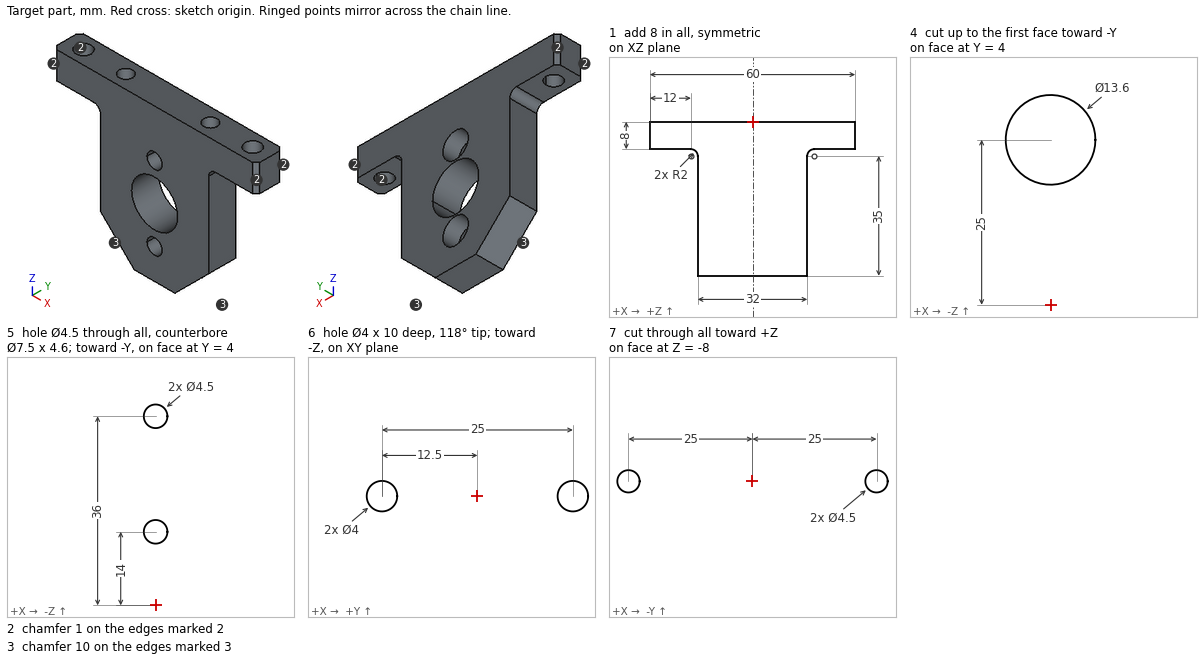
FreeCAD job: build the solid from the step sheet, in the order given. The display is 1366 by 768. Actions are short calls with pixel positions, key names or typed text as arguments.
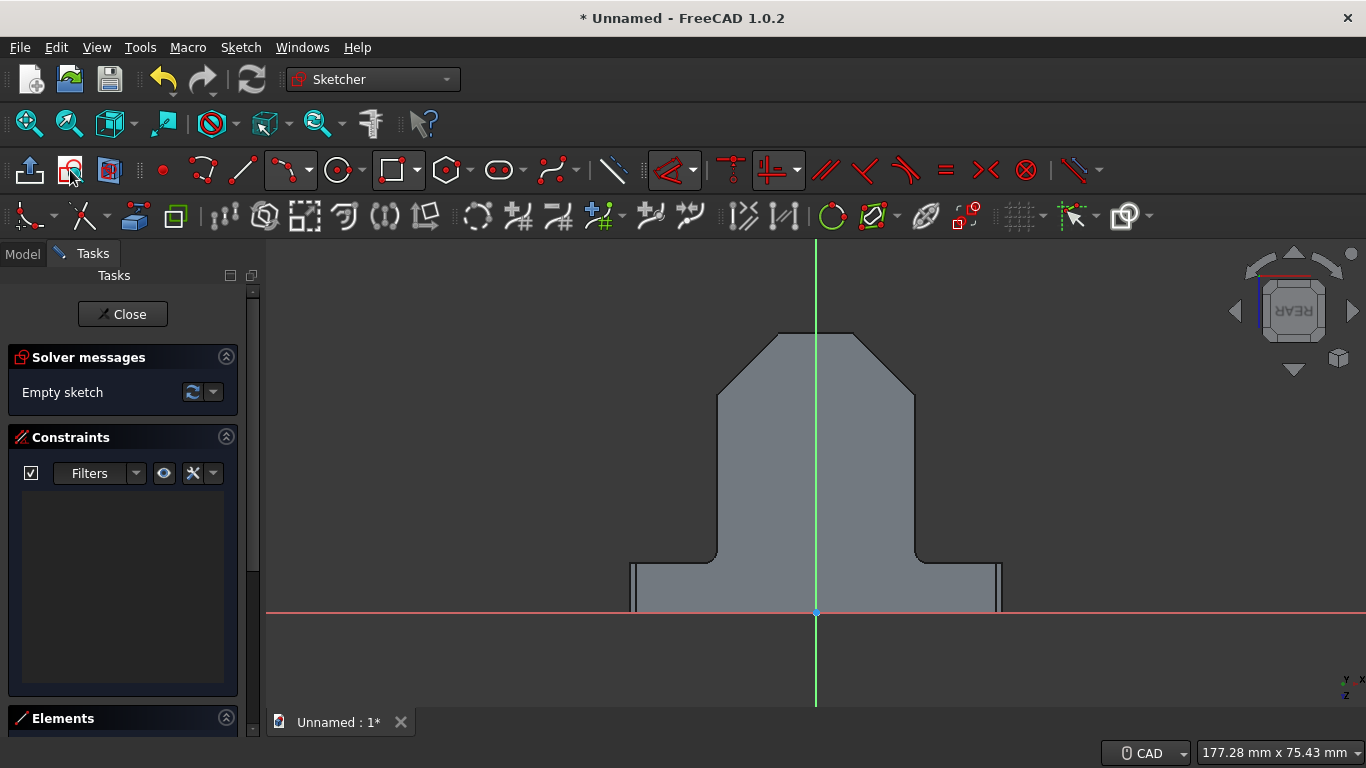
scroll(955, 597, up, 2)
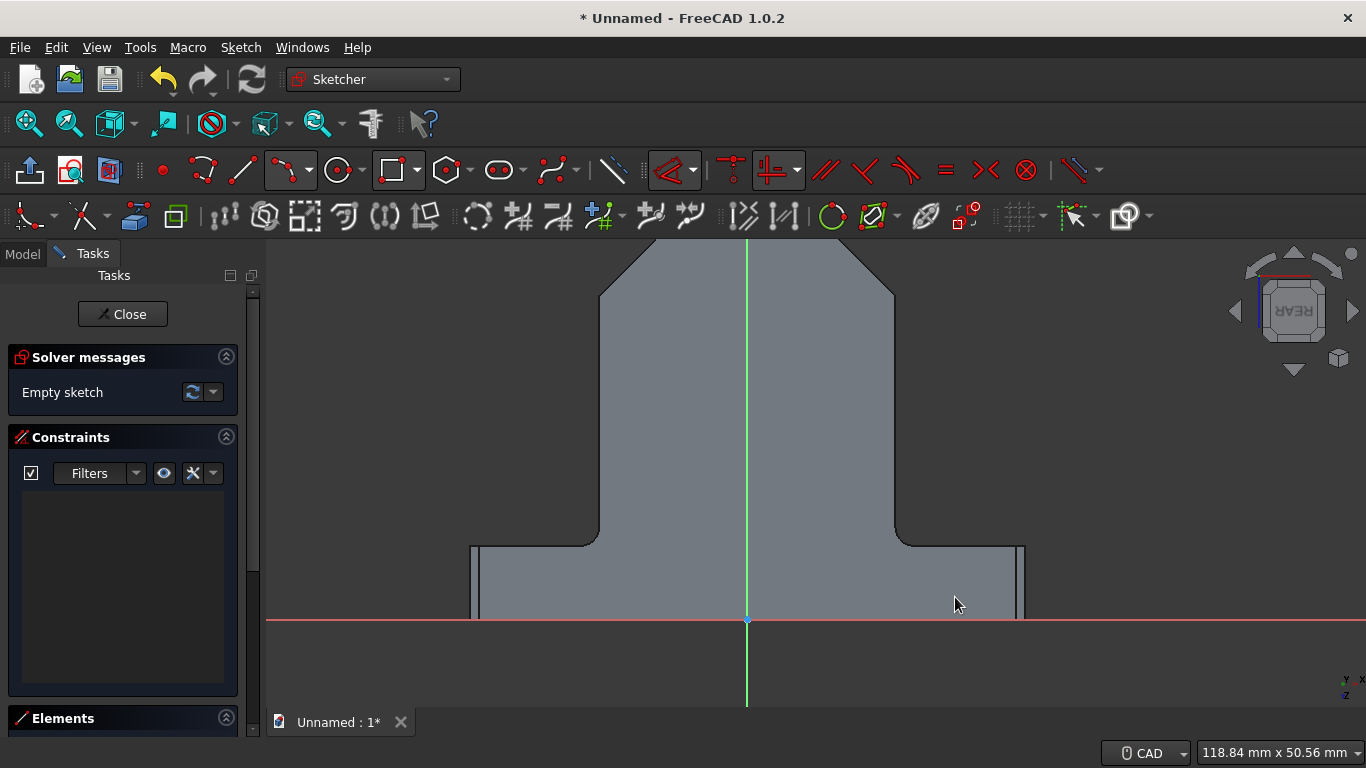
click(338, 170)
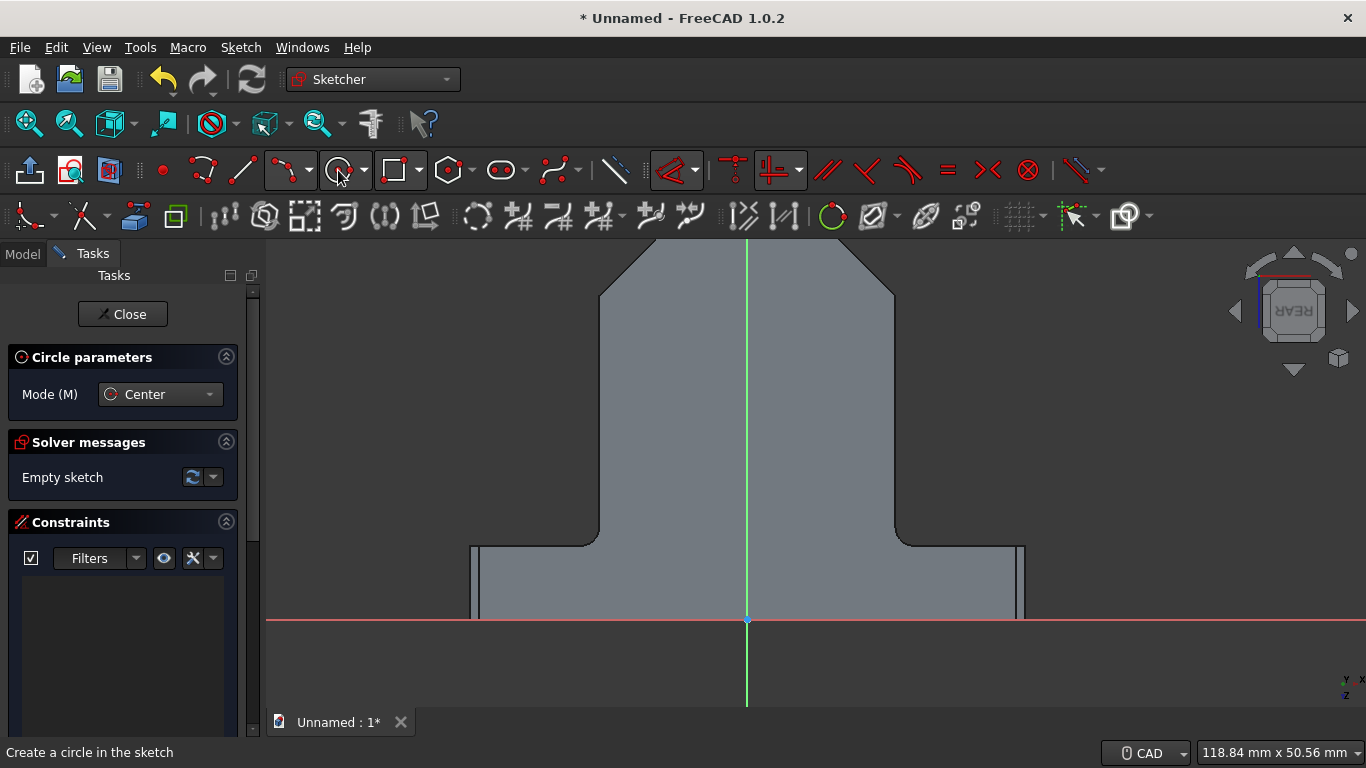
click(747, 388)
click(792, 344)
key(Escape)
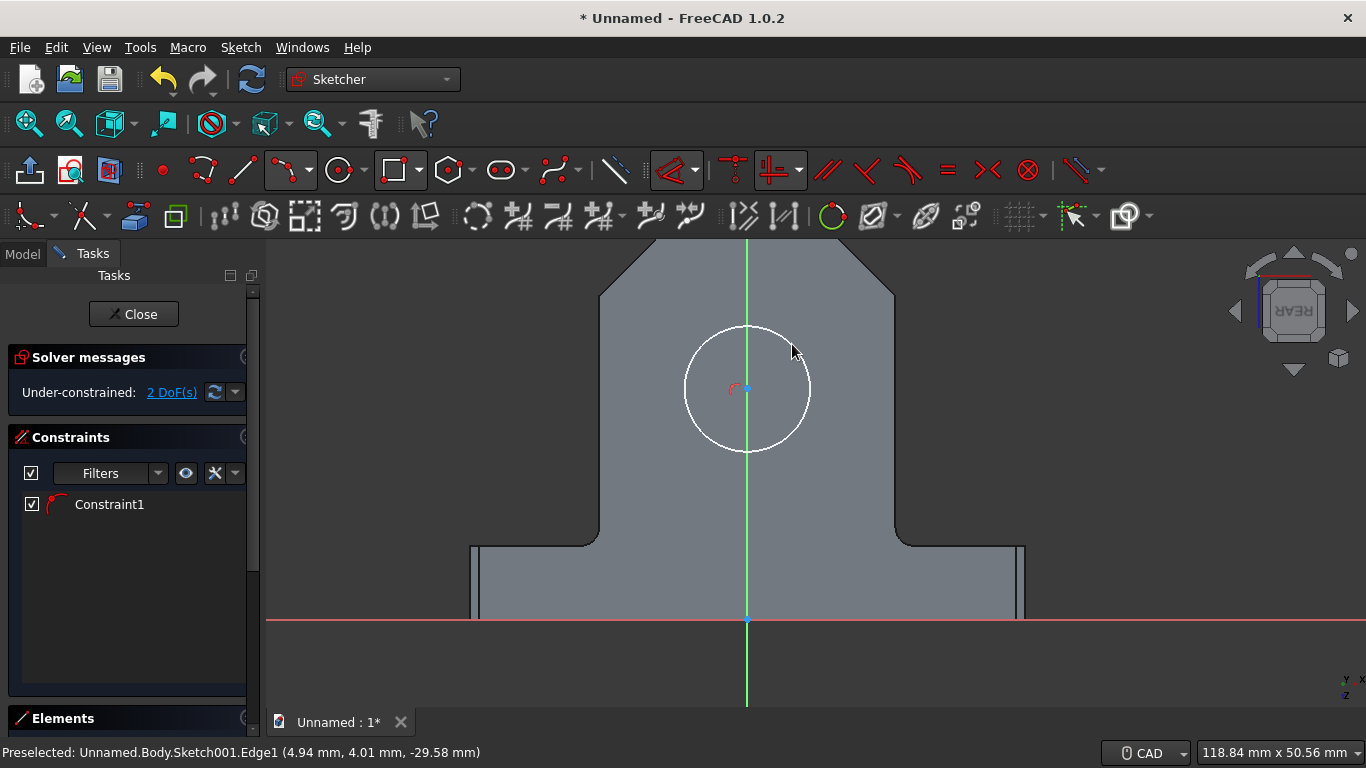
click(792, 345)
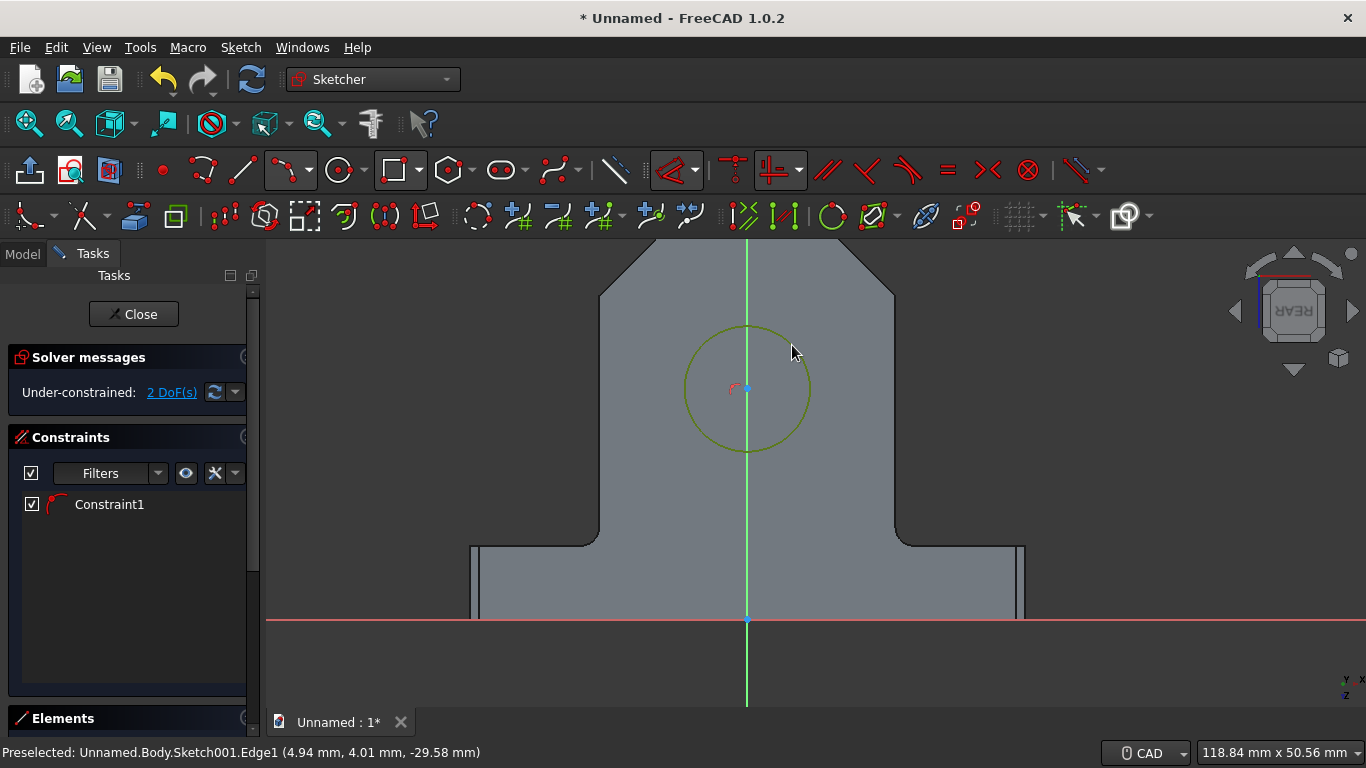
click(698, 170)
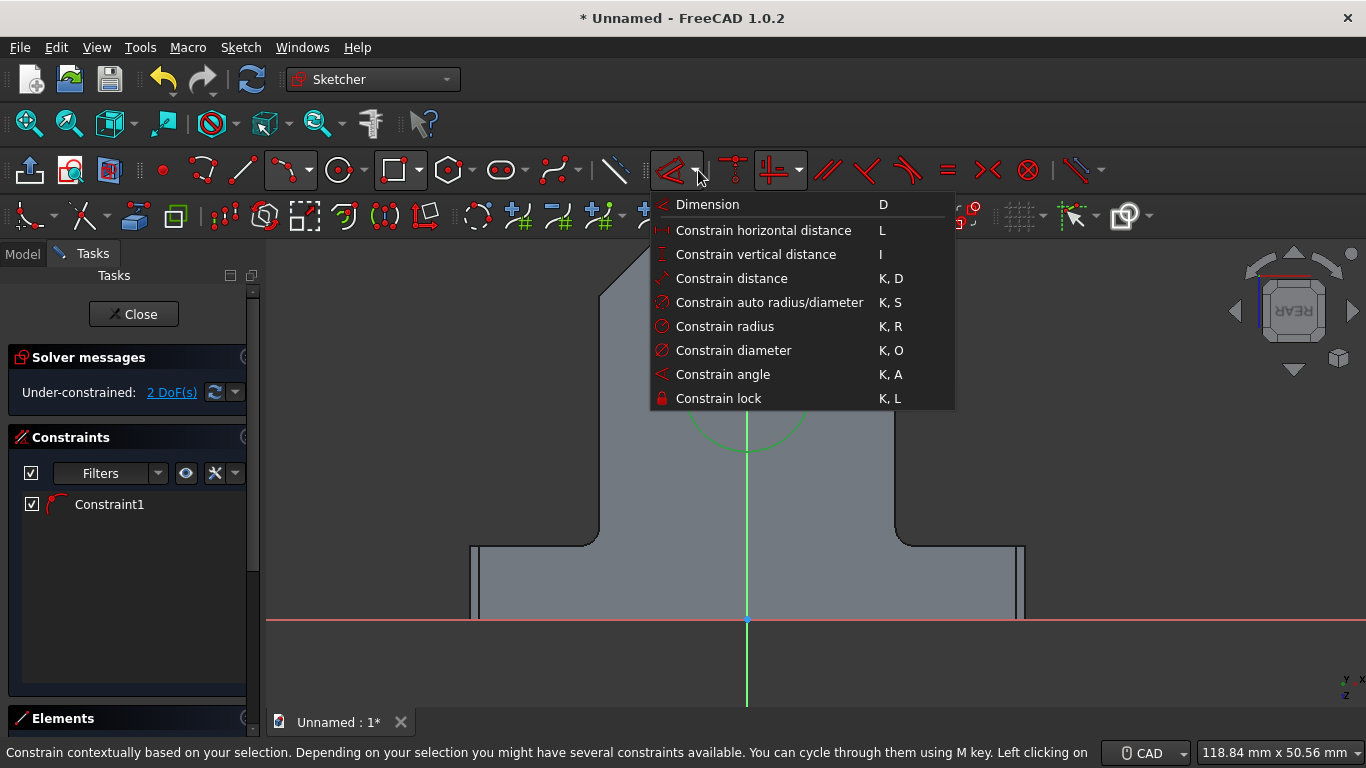
click(803, 350)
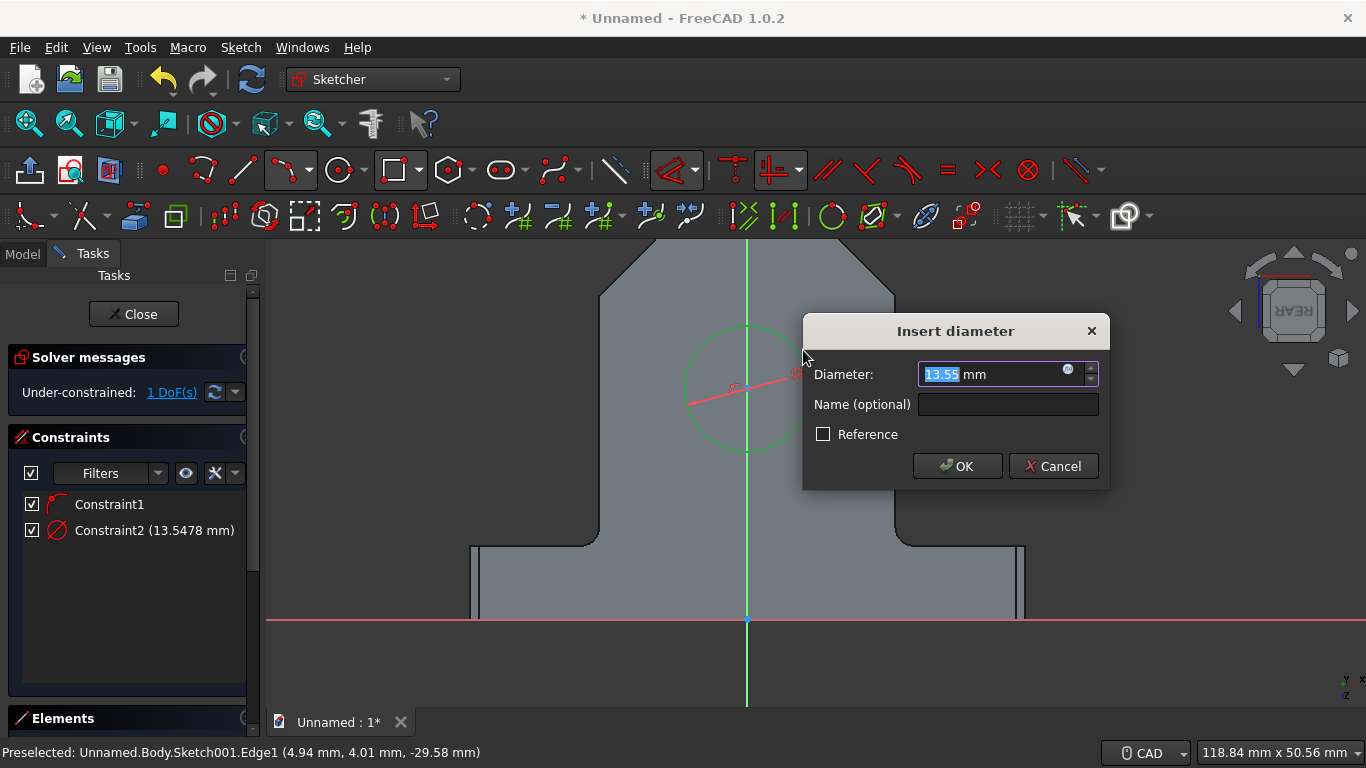
text(13.6)
key(Return)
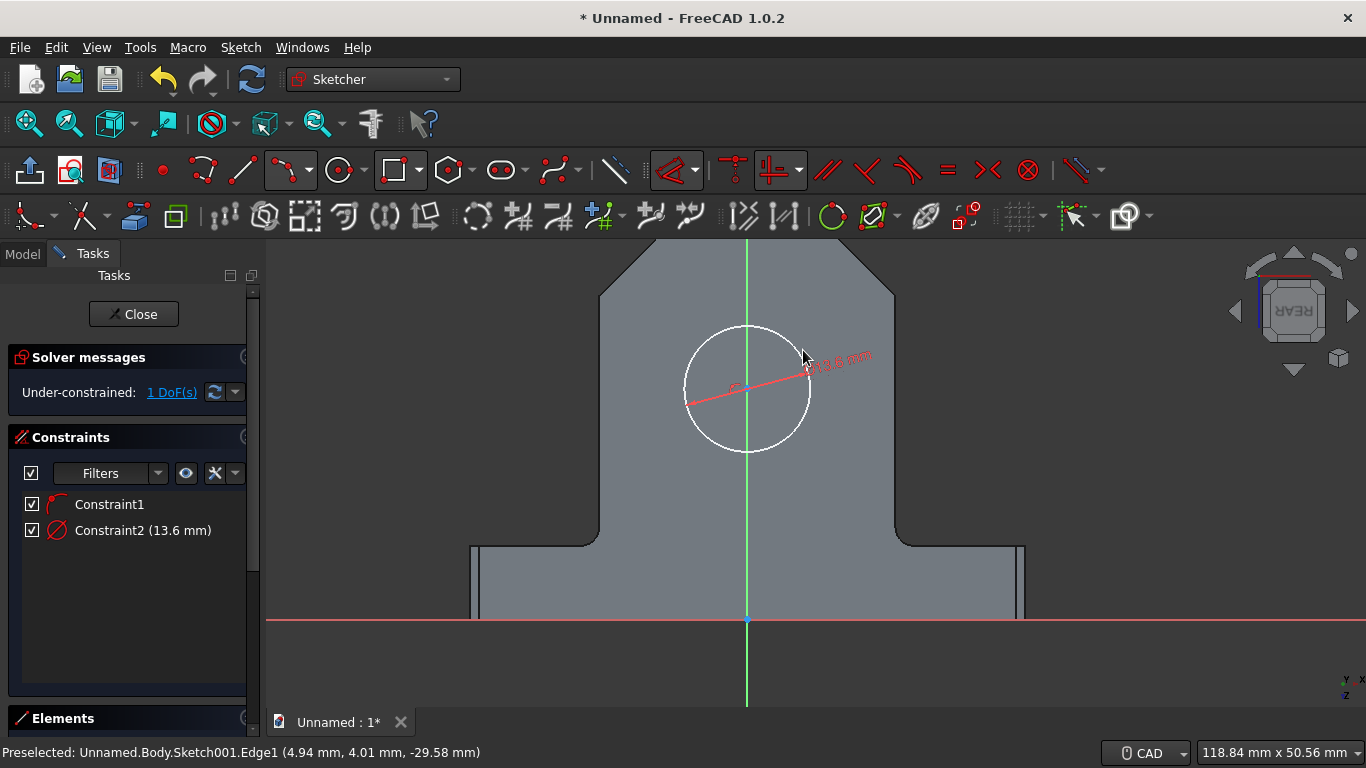
click(747, 389)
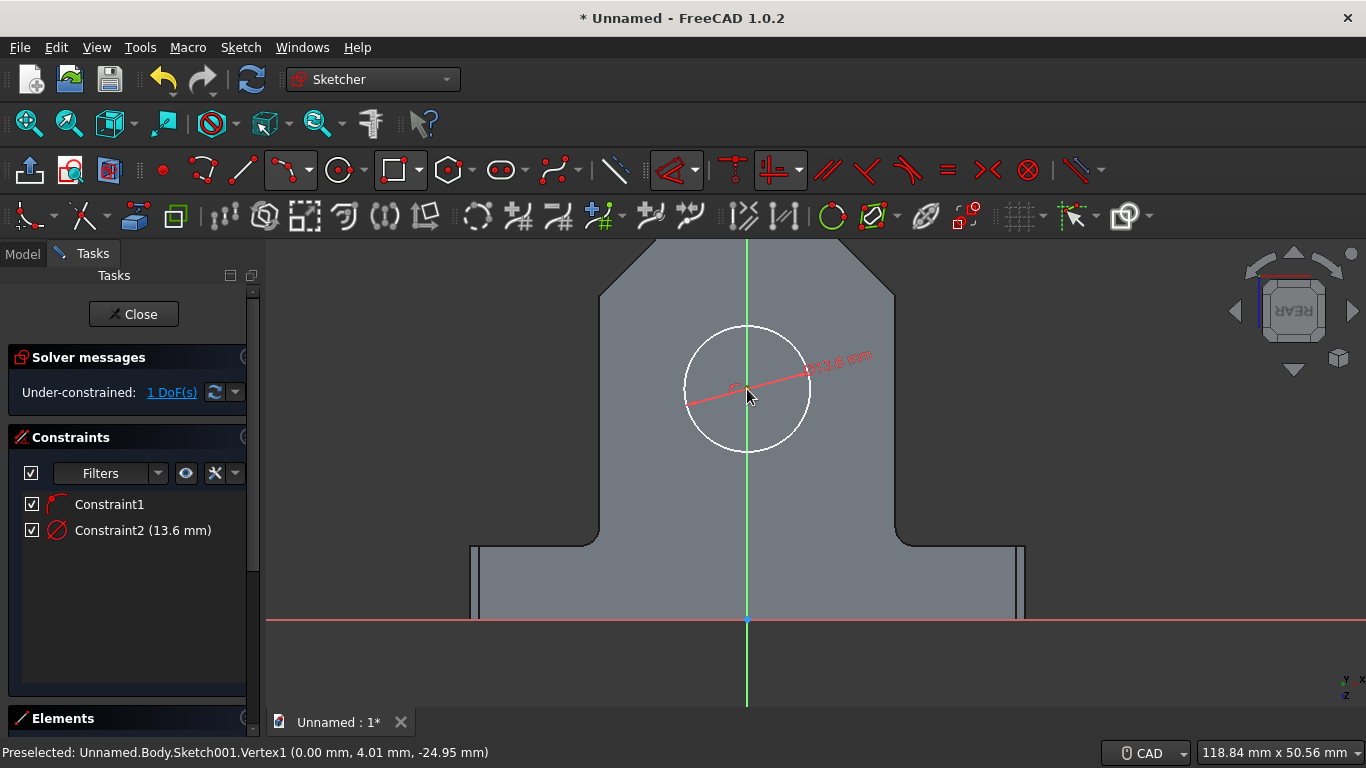
key(i)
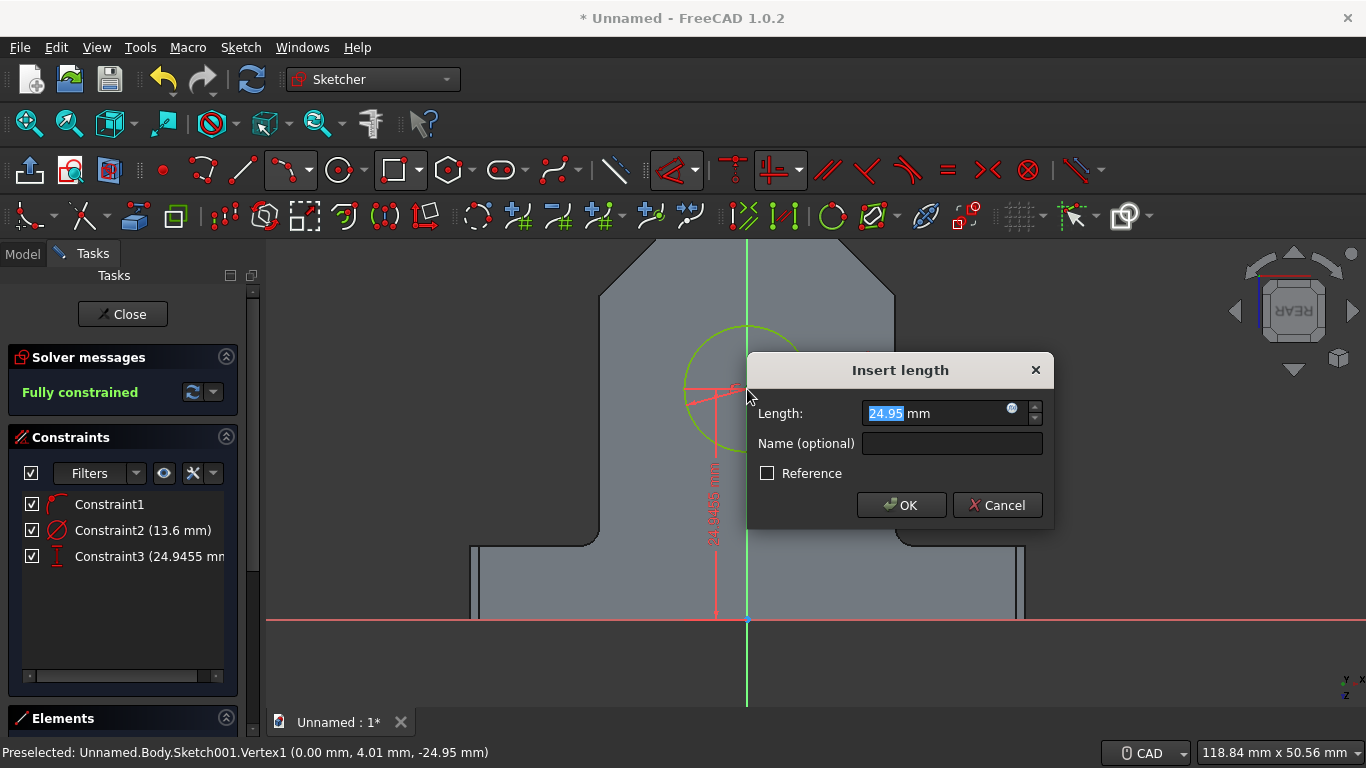
text(25)
key(Return)